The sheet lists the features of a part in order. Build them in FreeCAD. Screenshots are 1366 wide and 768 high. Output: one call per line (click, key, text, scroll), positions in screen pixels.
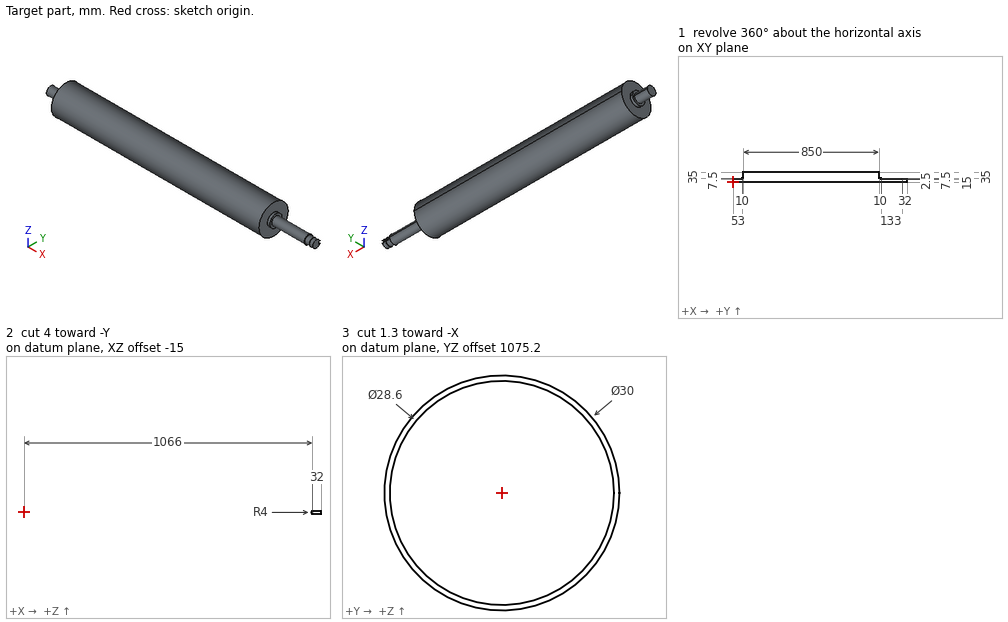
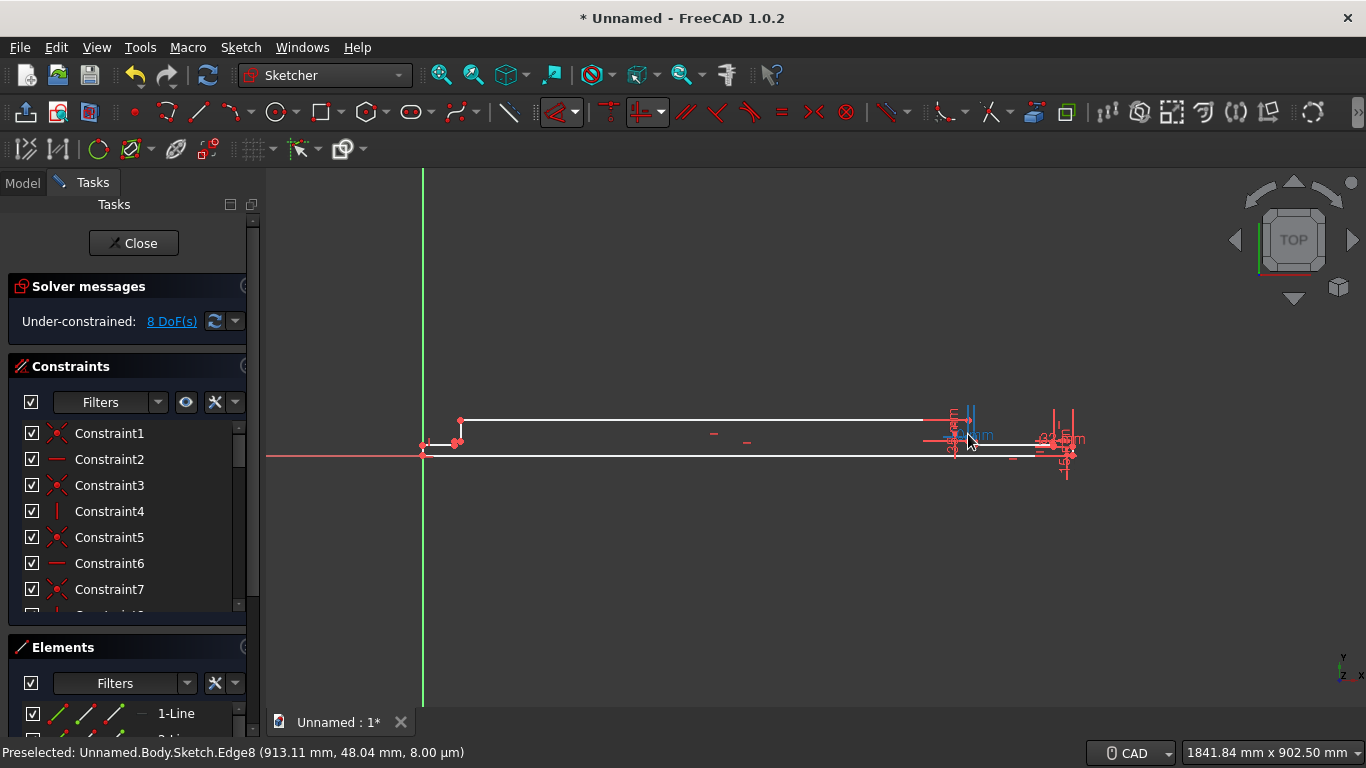
scroll(461, 427, up, 4)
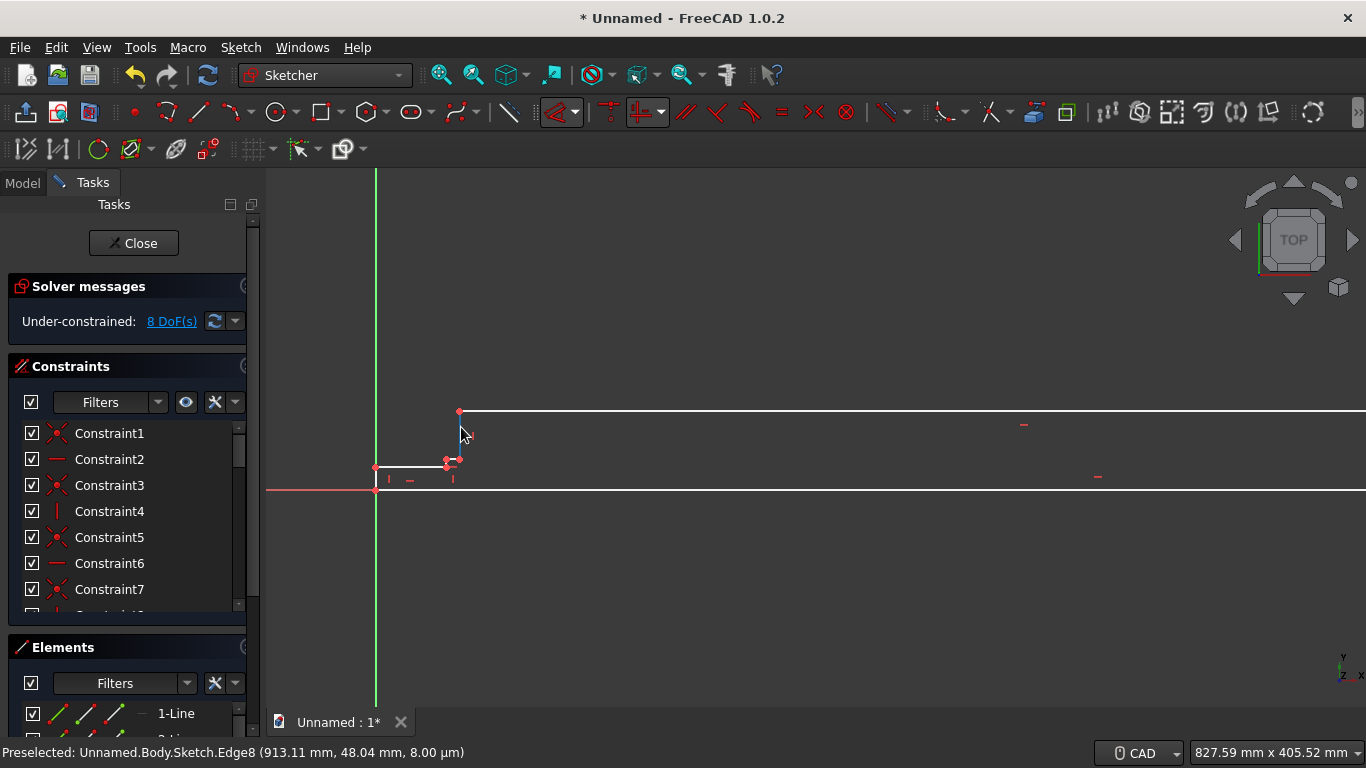
click(460, 426)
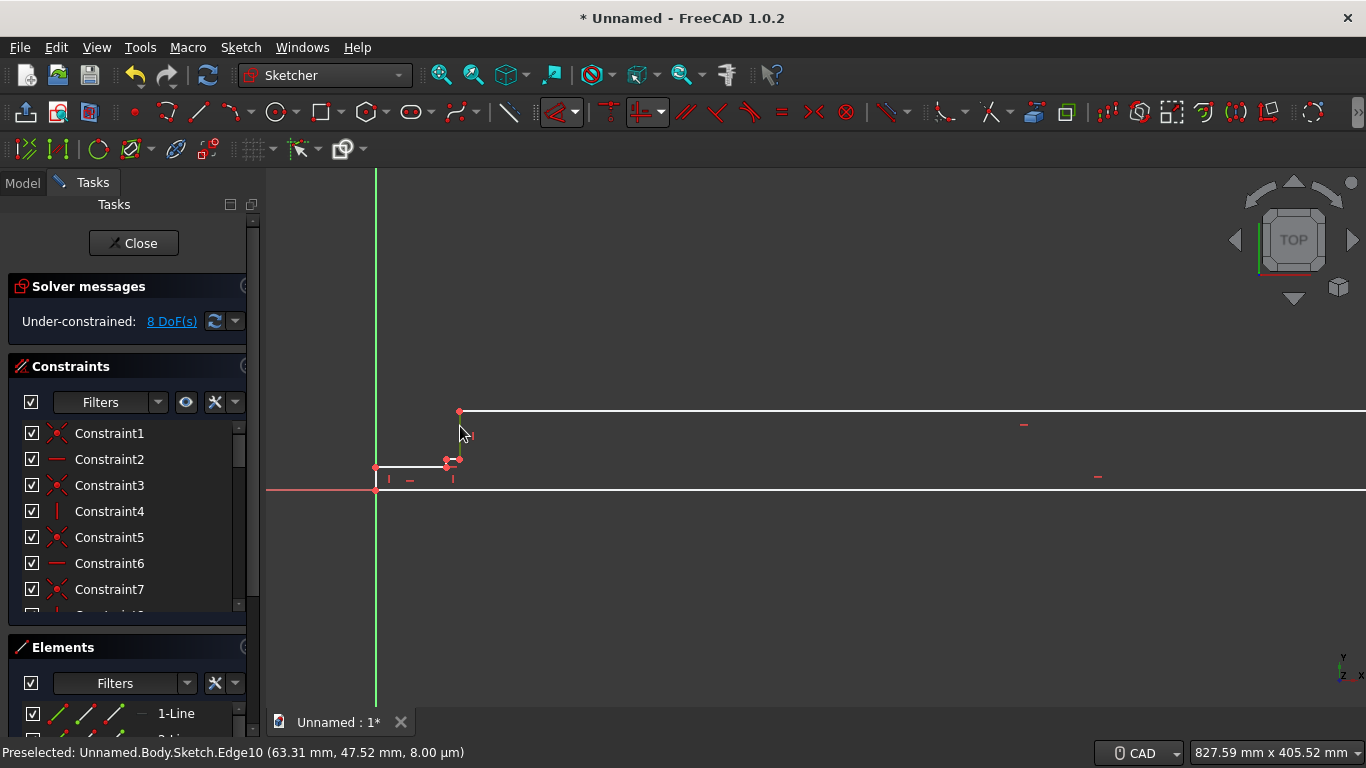
key(i)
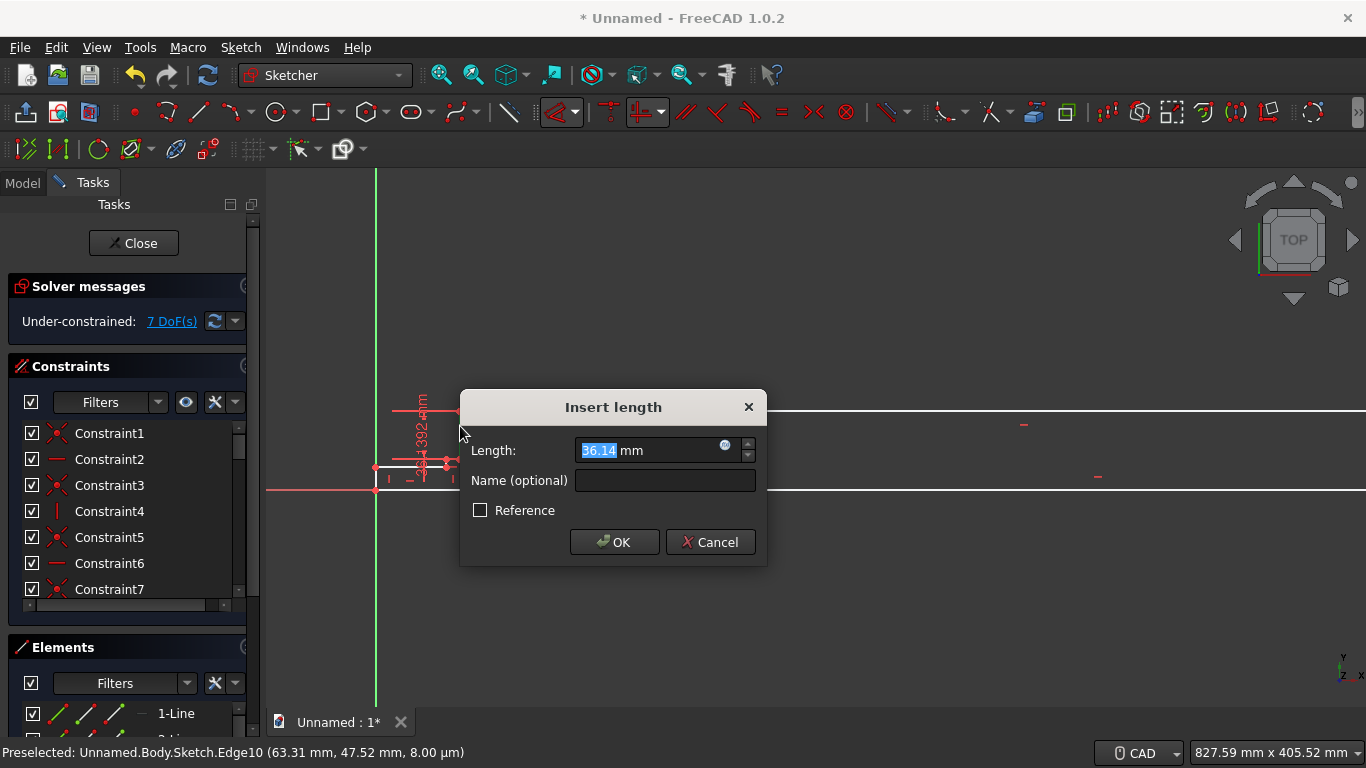
text(35)
key(Return)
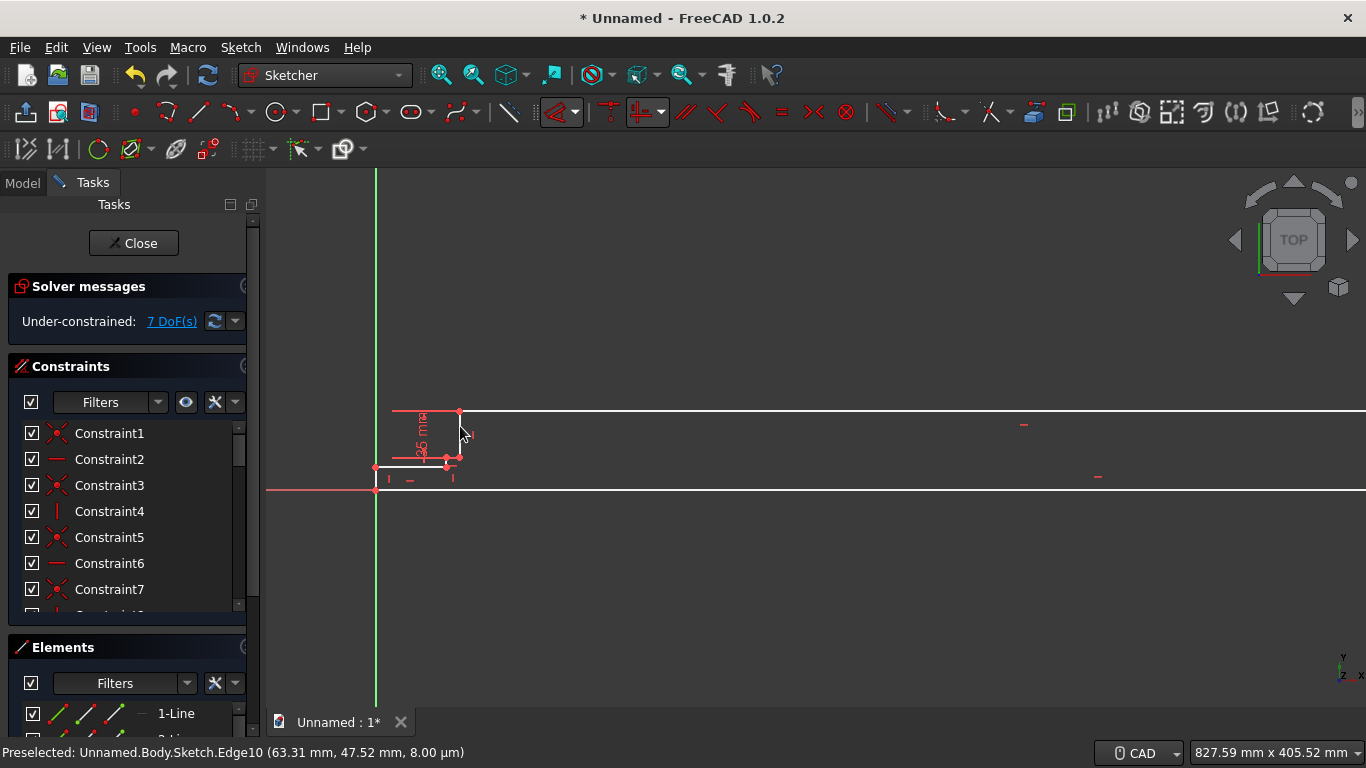
scroll(453, 458, up, 6)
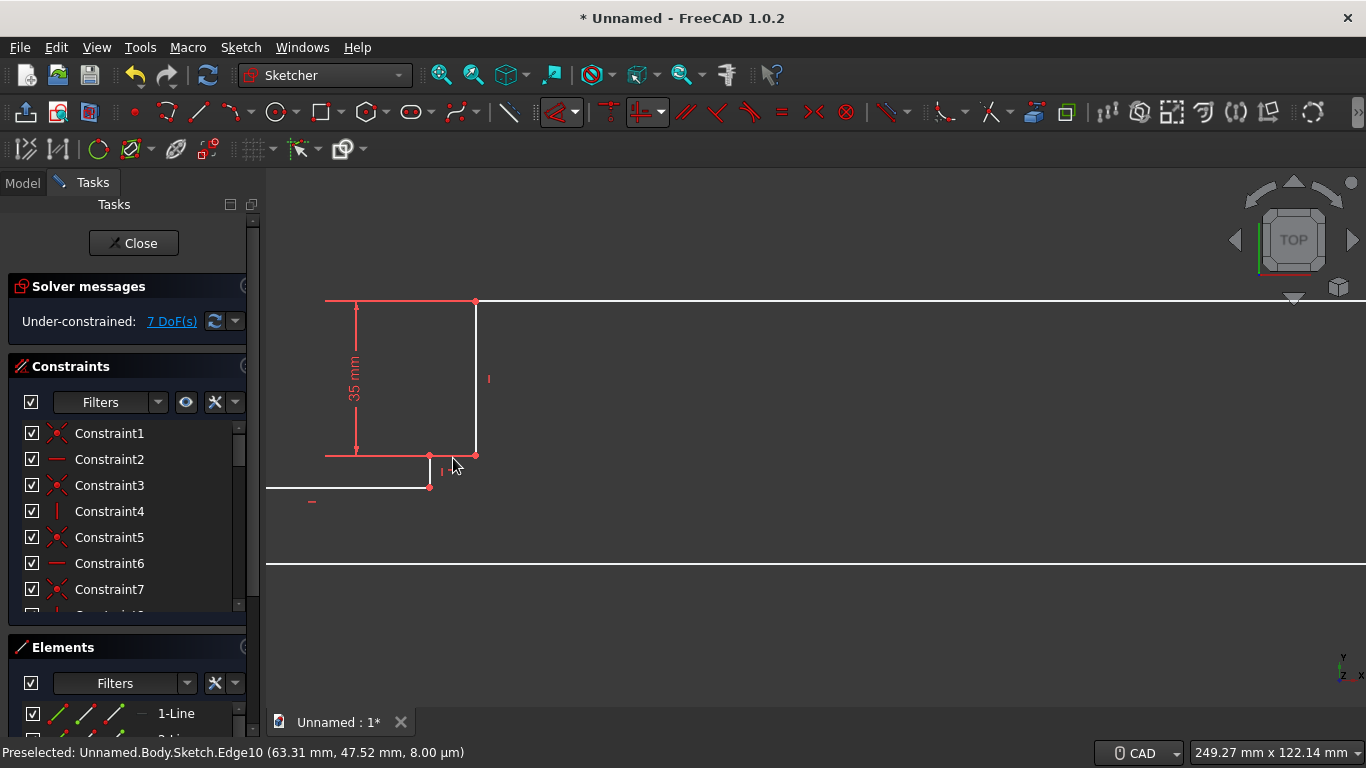
click(453, 456)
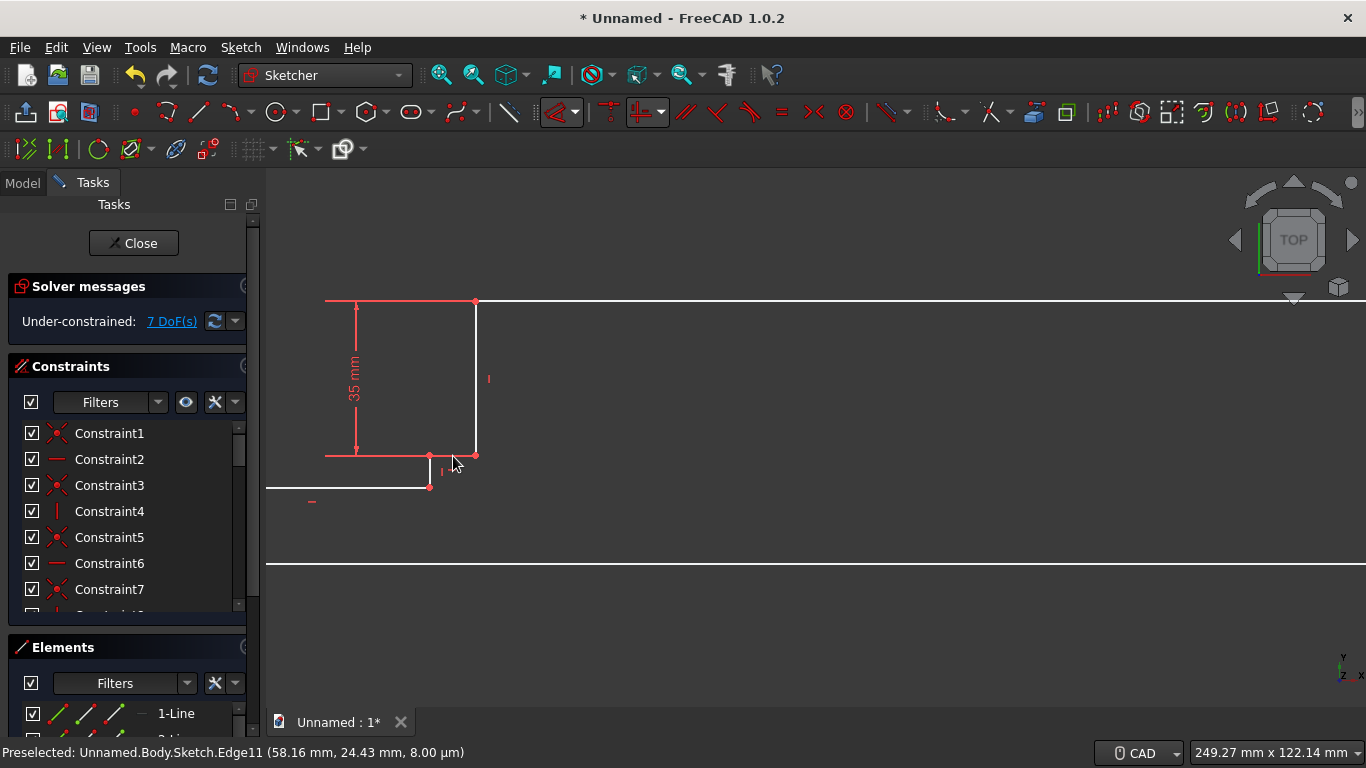
key(l)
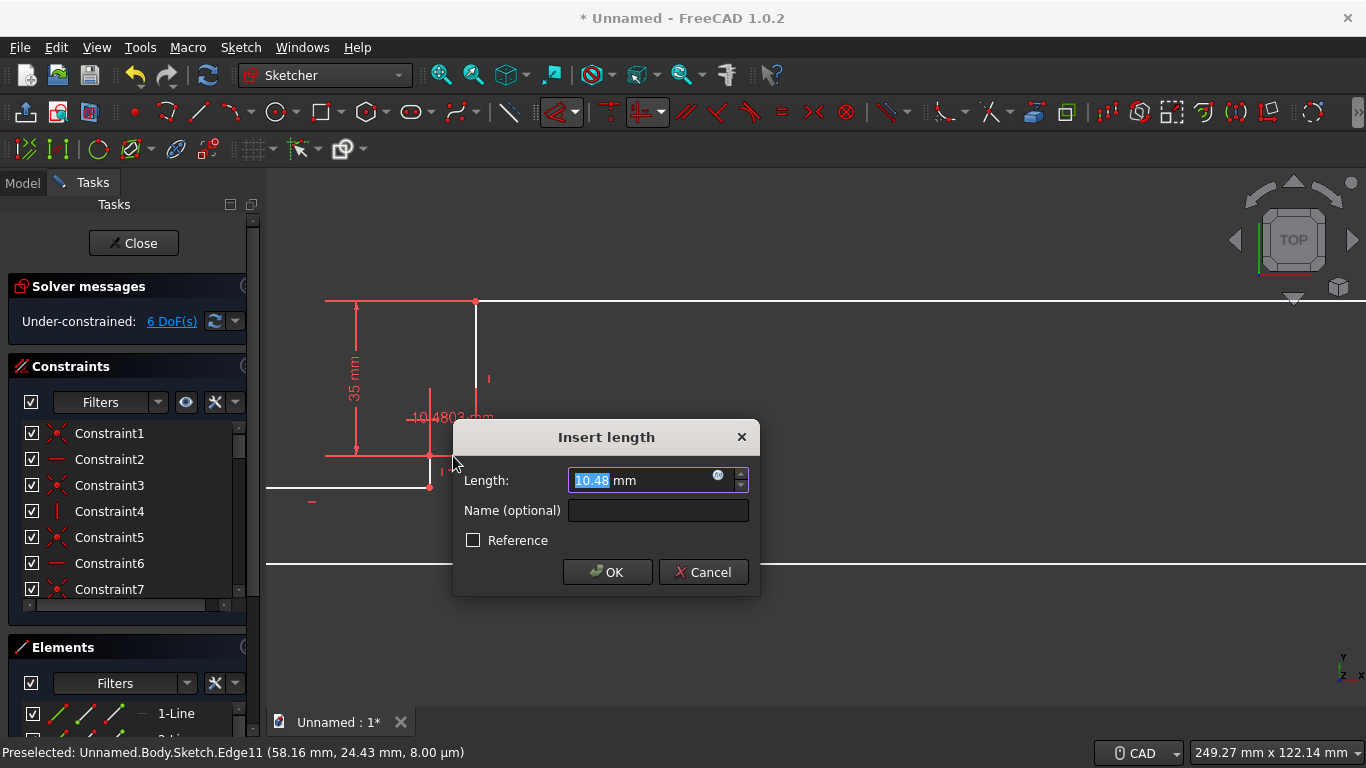
text(10)
key(Return)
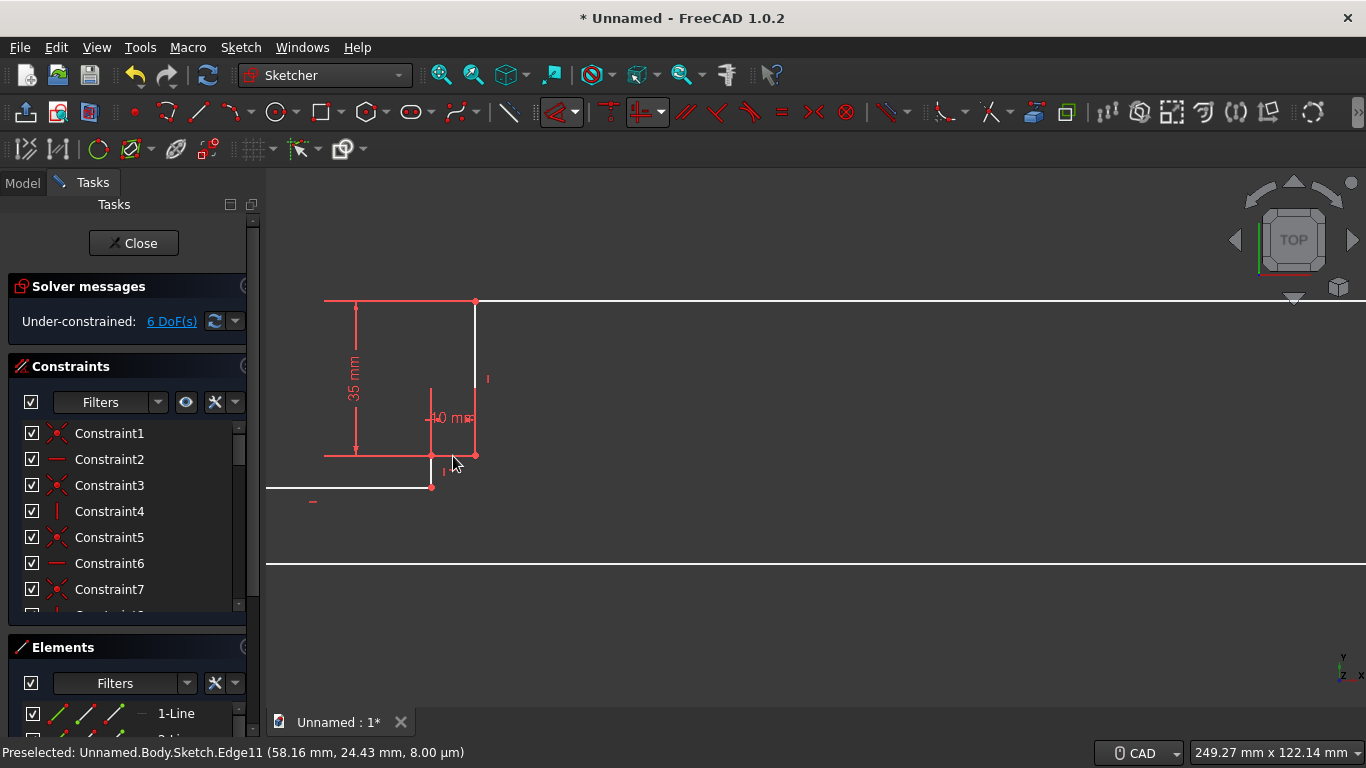
scroll(458, 438, down, 10)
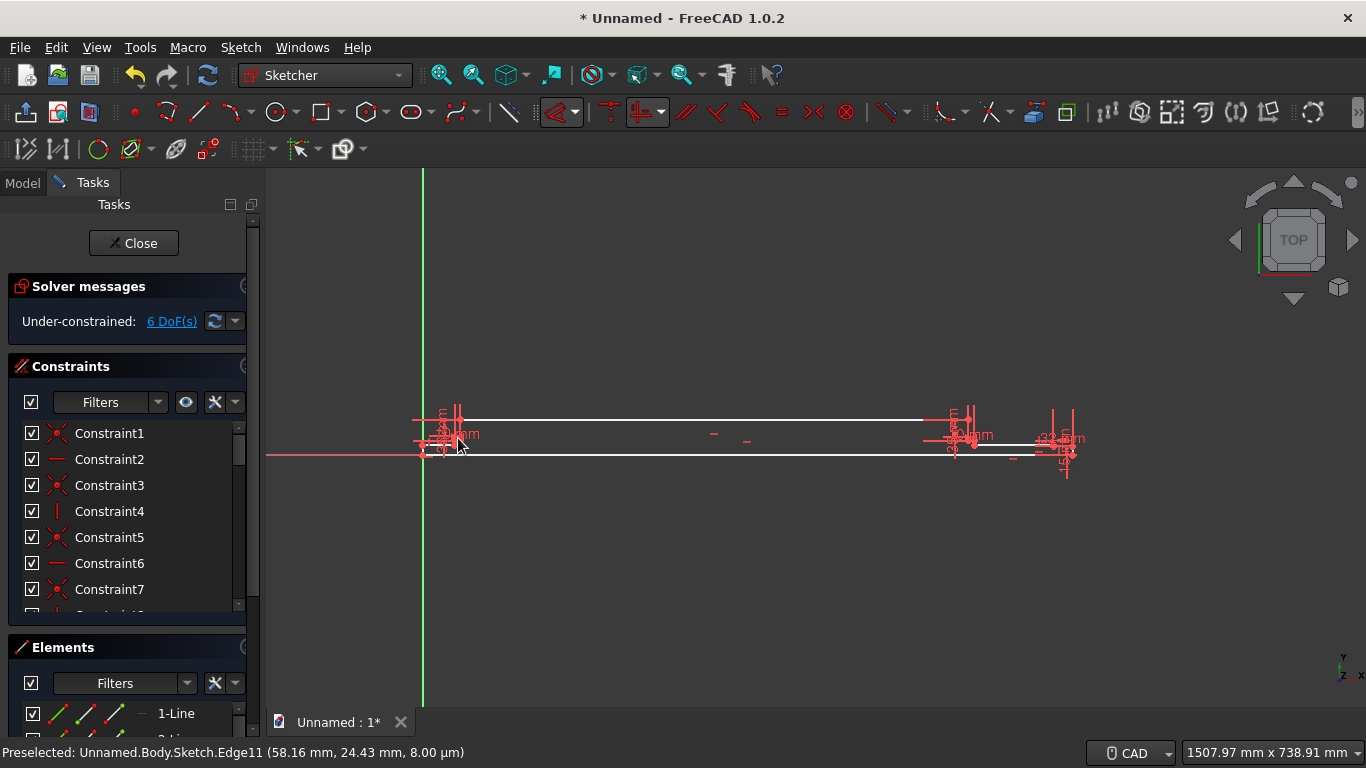
scroll(445, 445, up, 2)